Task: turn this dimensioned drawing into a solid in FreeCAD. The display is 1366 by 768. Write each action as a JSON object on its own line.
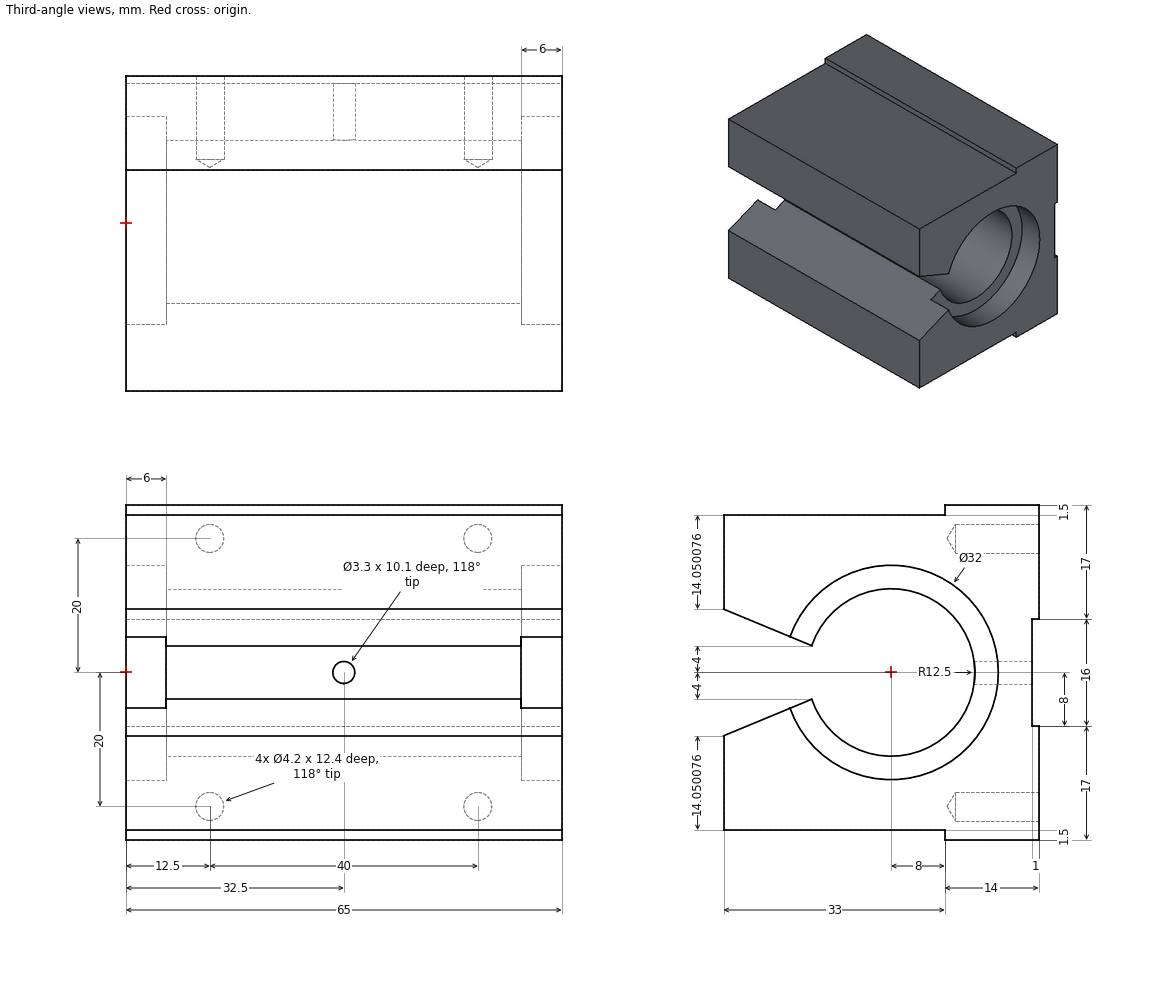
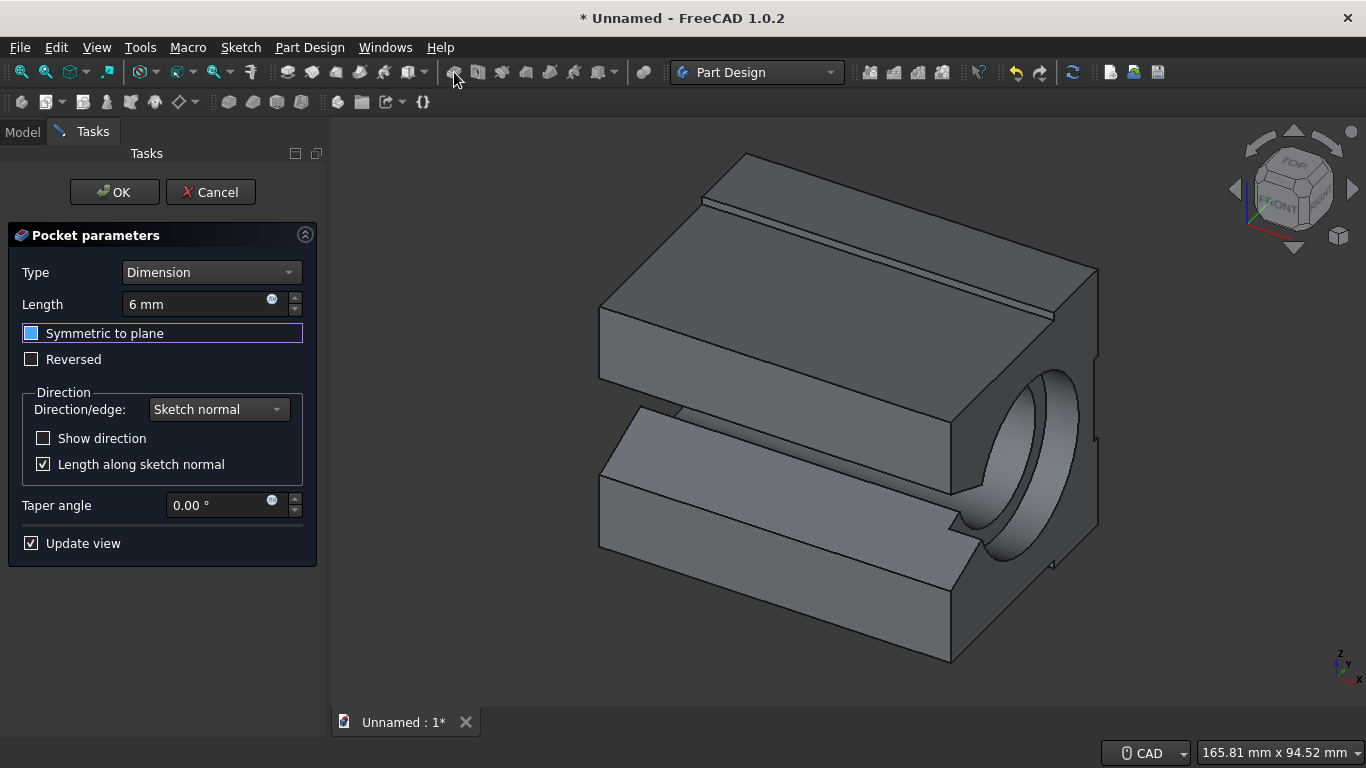
{"action": "left_click", "coordinate": [115, 192]}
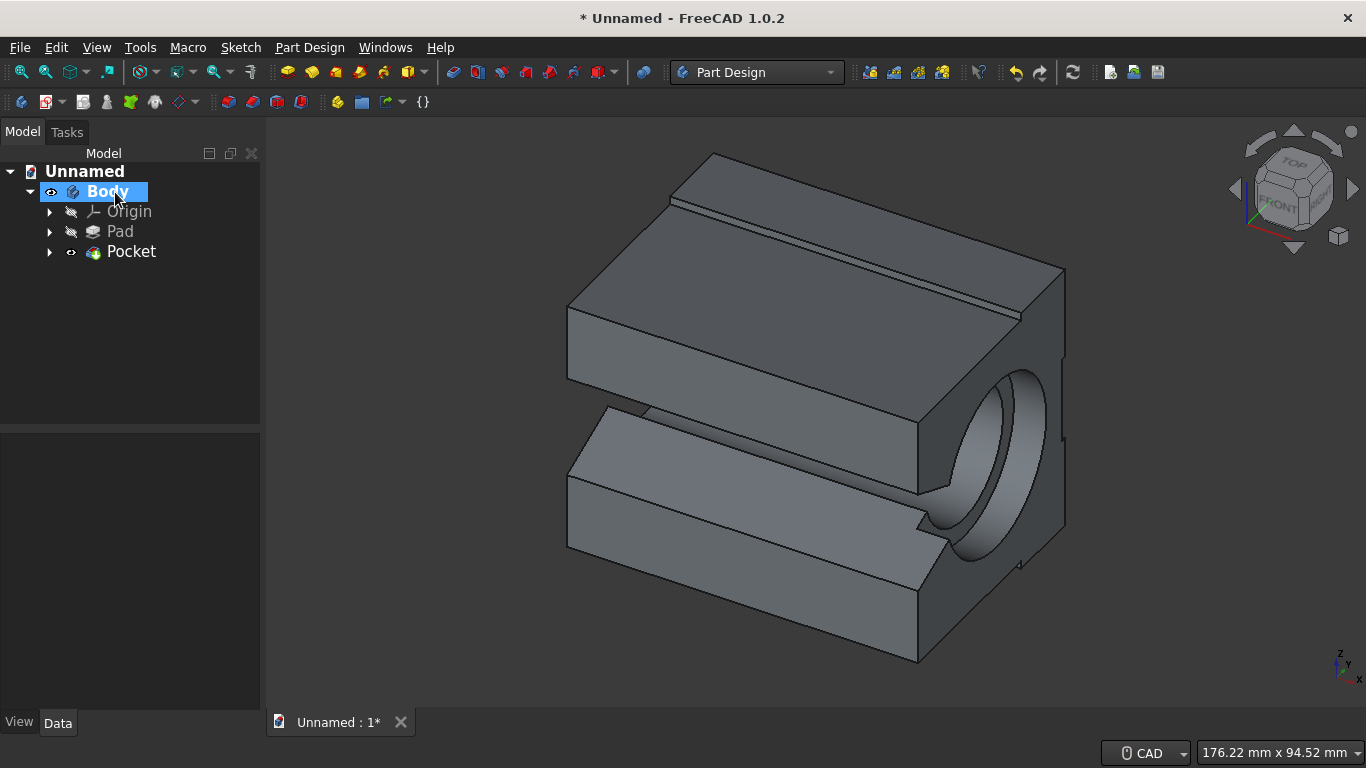
{"action": "left_click", "coordinate": [50, 212]}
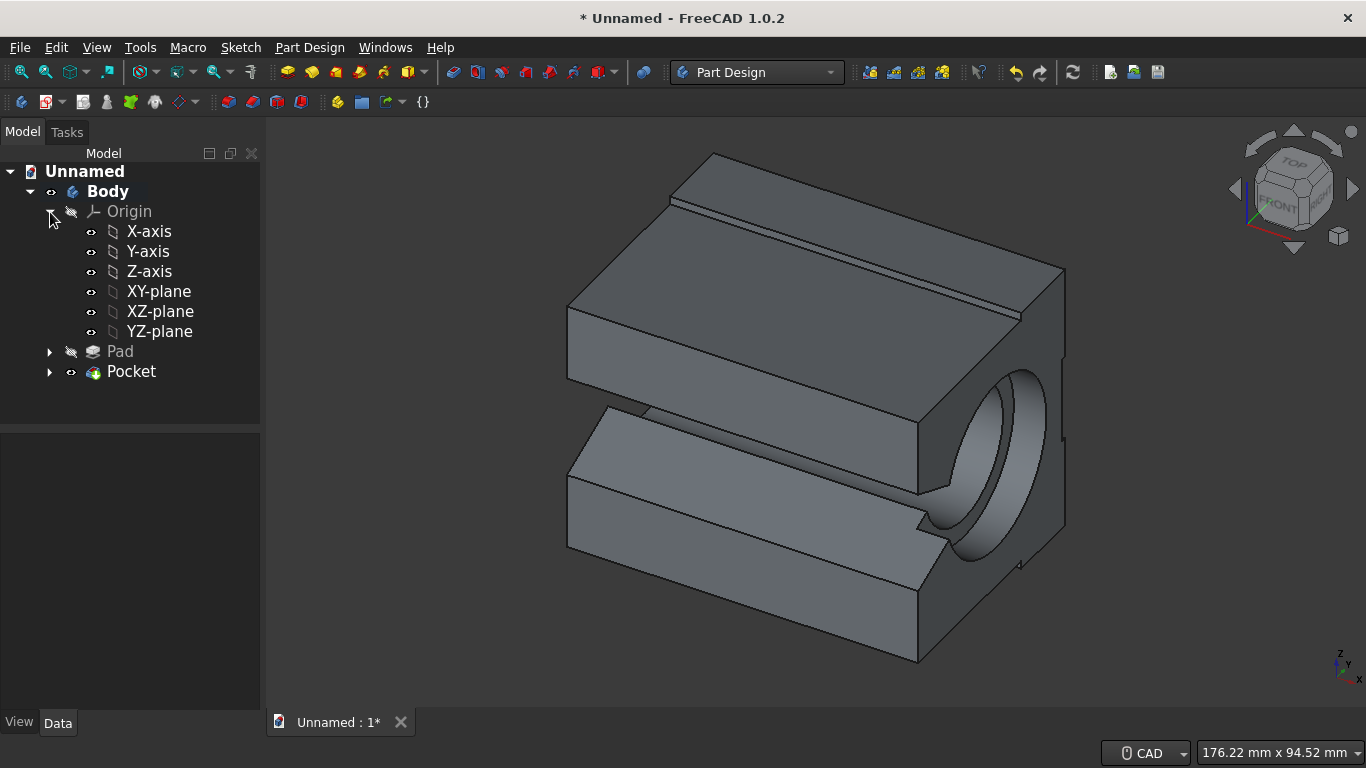
{"action": "left_click", "coordinate": [136, 332]}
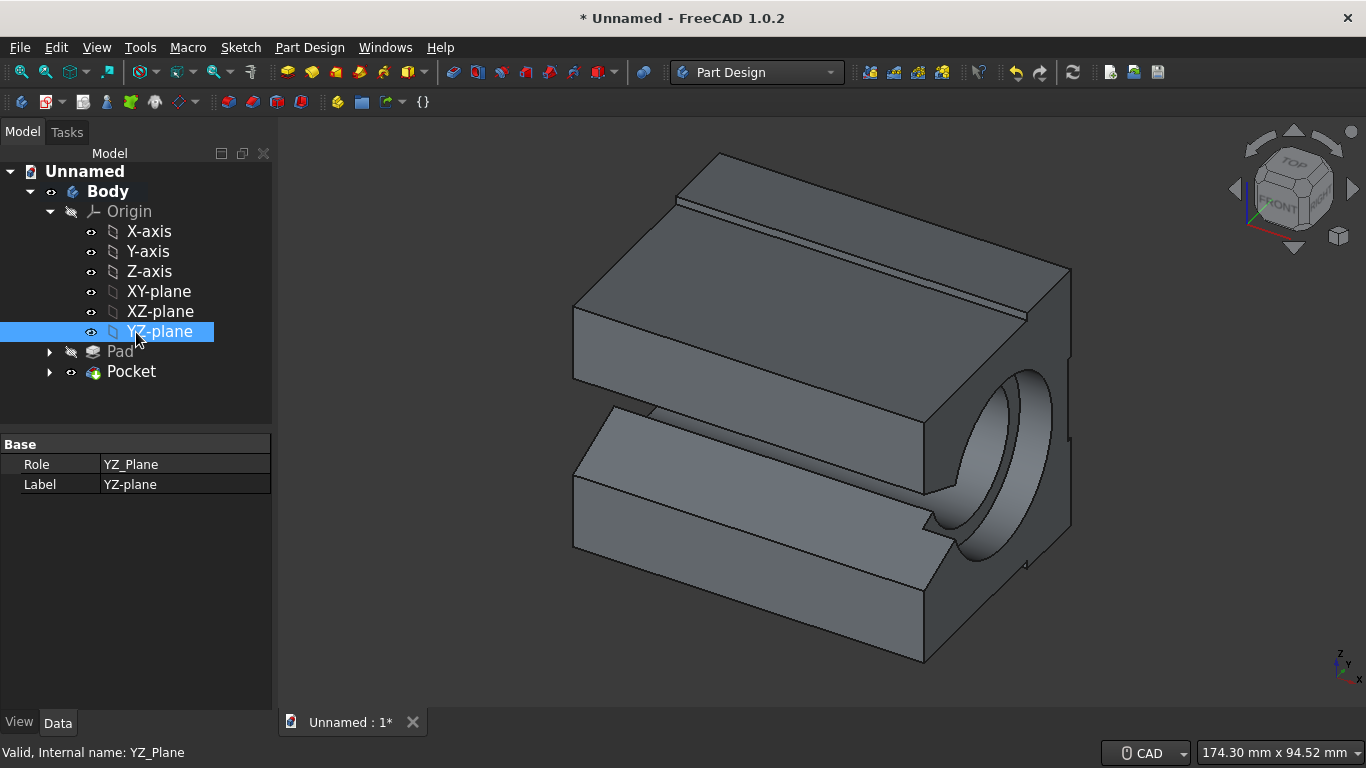
{"action": "left_click", "coordinate": [180, 102]}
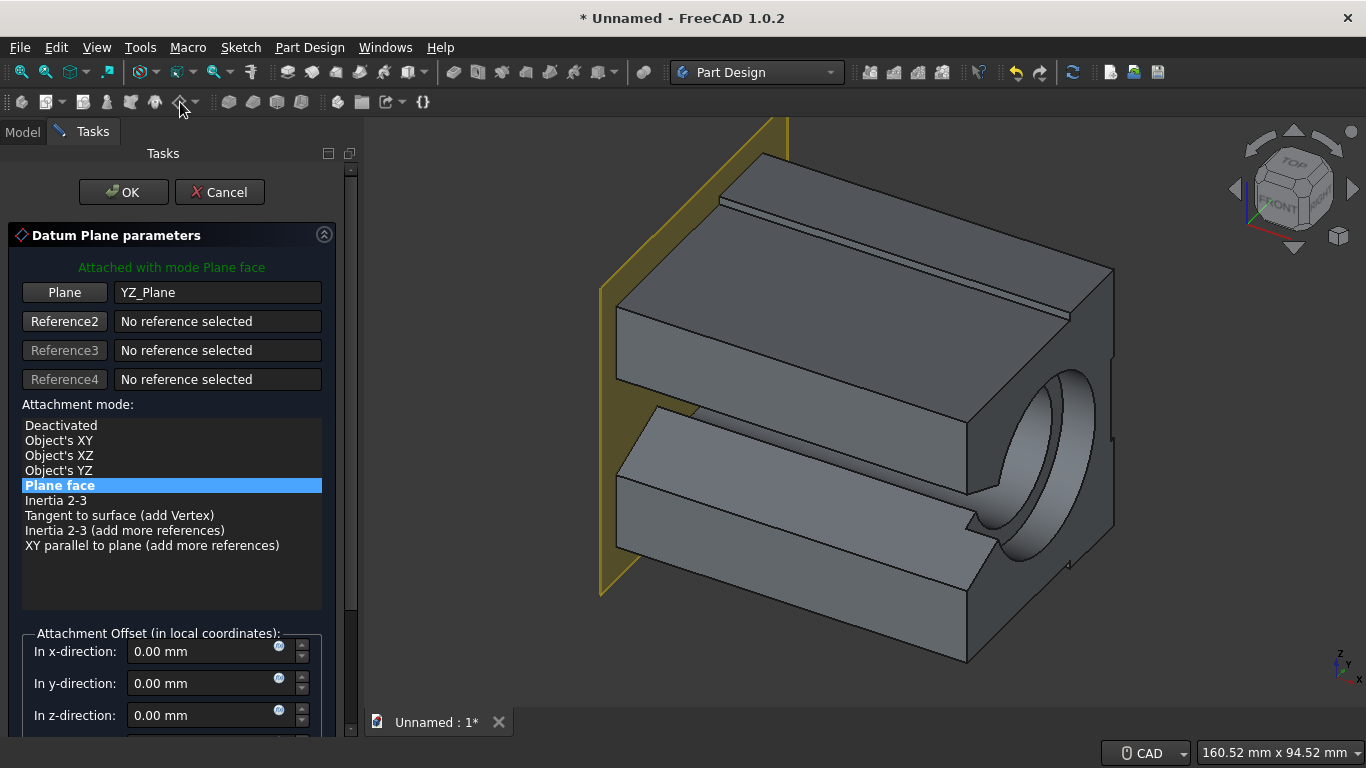
{"action": "triple_click", "coordinate": [210, 715]}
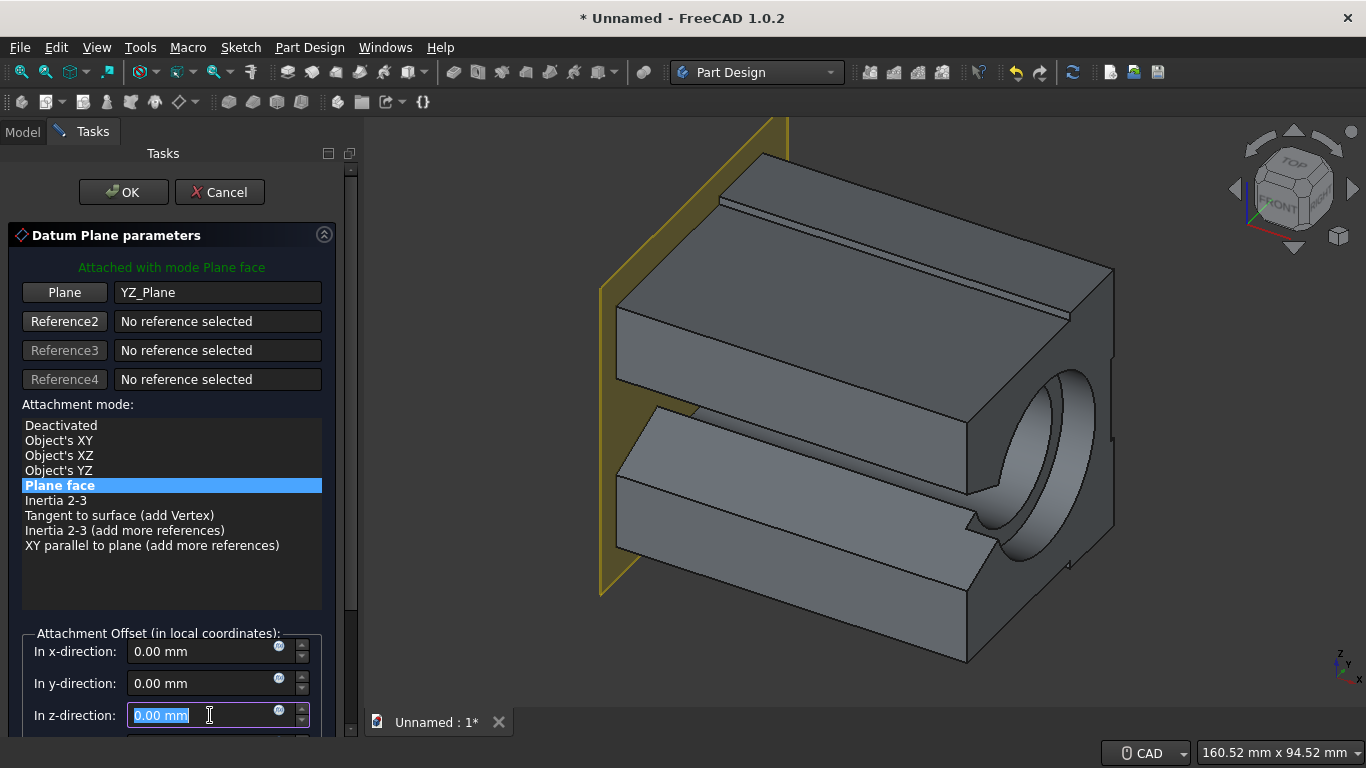
{"action": "type", "text": "6"}
{"action": "key", "text": "Tab"}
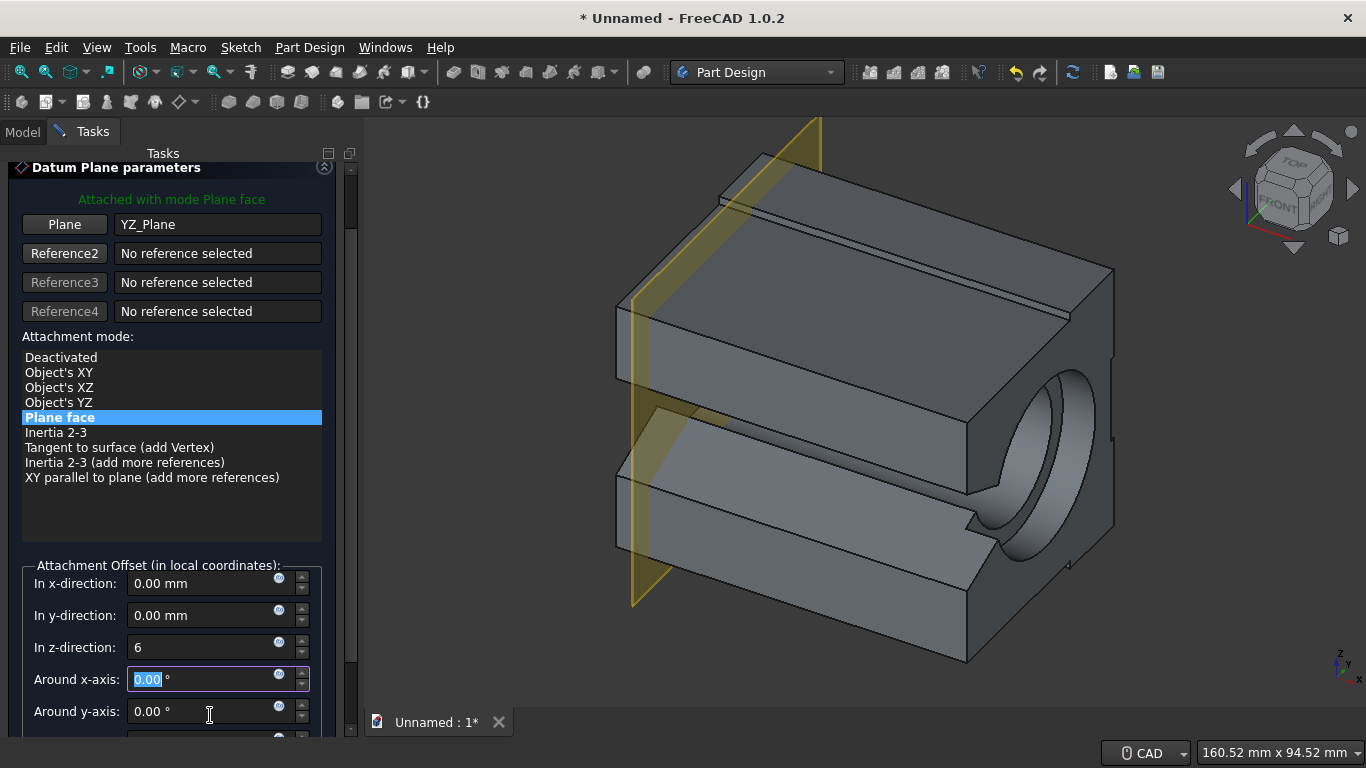
{"action": "scroll", "coordinate": [351, 450], "scroll_direction": "up", "scroll_amount": 2}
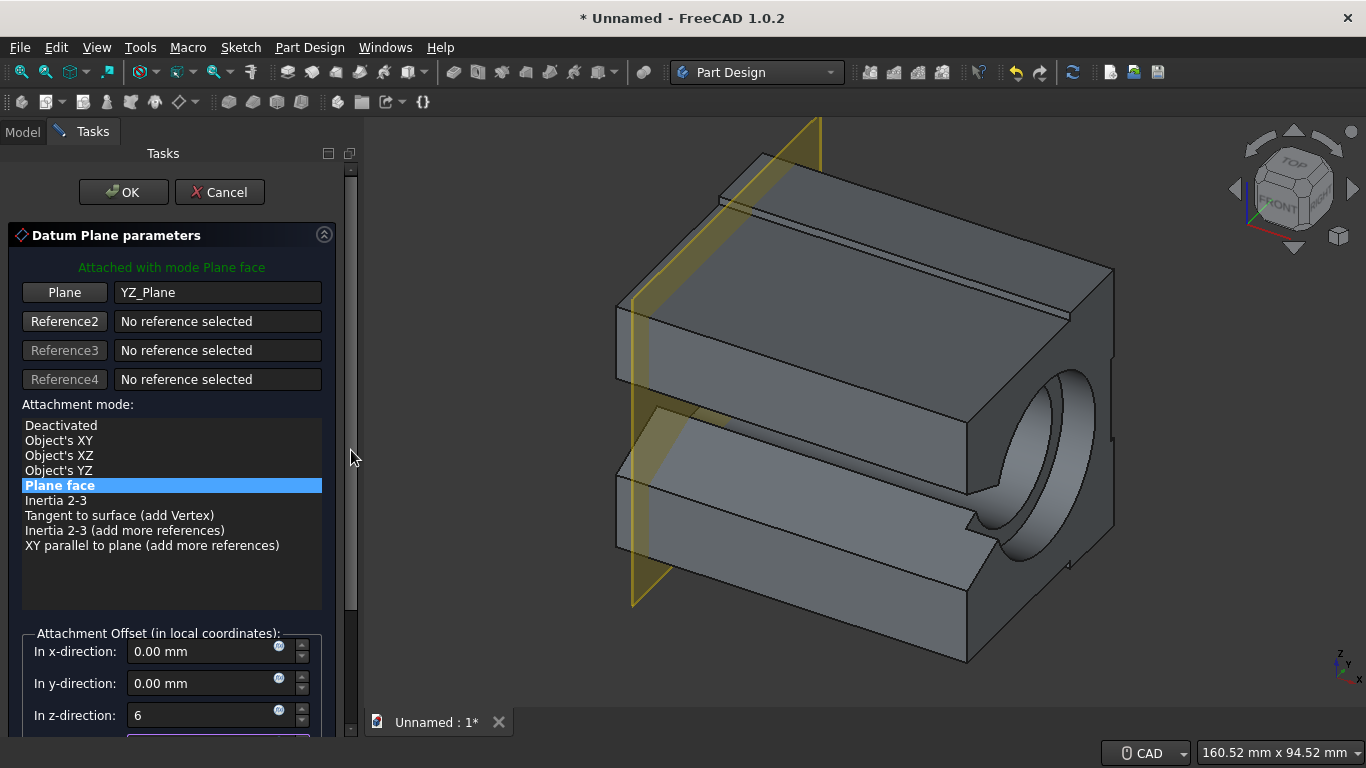
{"action": "left_click", "coordinate": [124, 192]}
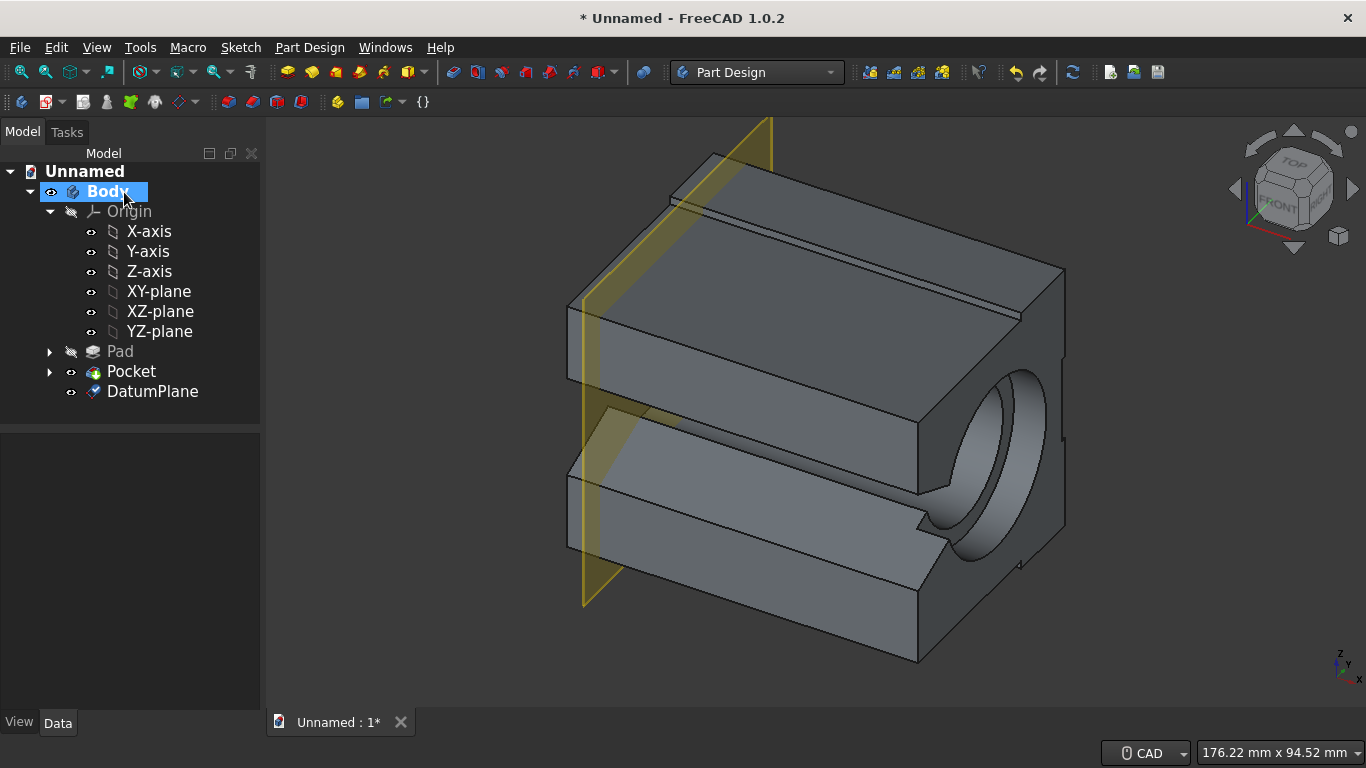
{"action": "left_click", "coordinate": [116, 392]}